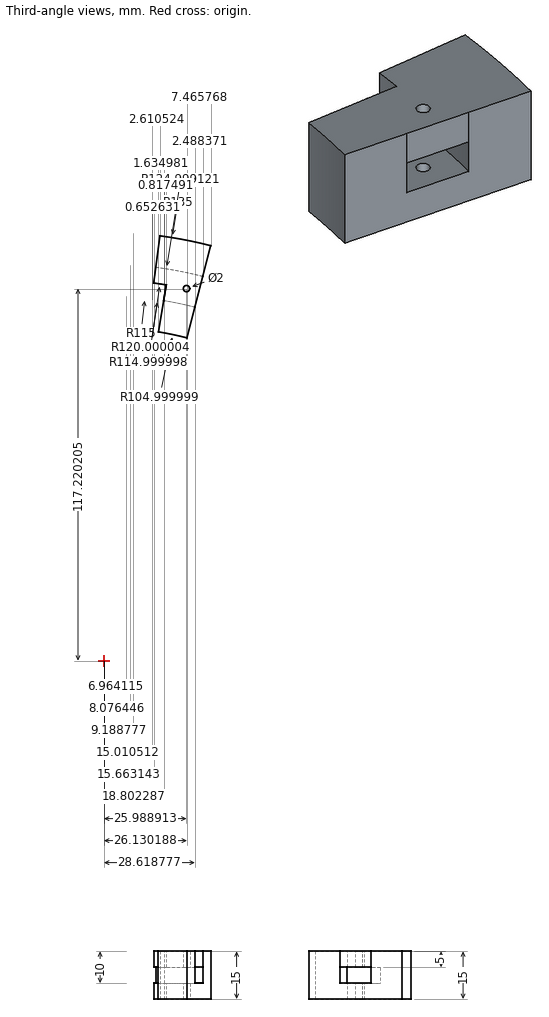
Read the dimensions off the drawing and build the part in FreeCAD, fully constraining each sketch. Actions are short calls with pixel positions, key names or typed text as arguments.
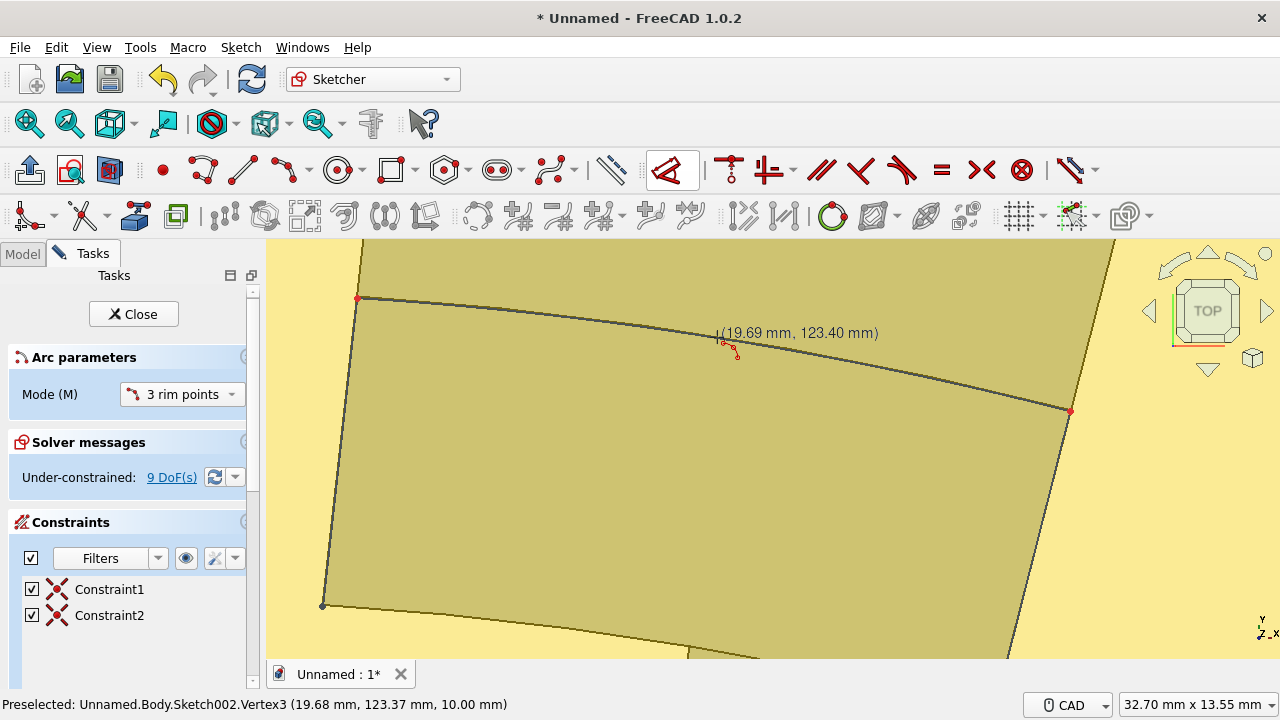
click(323, 607)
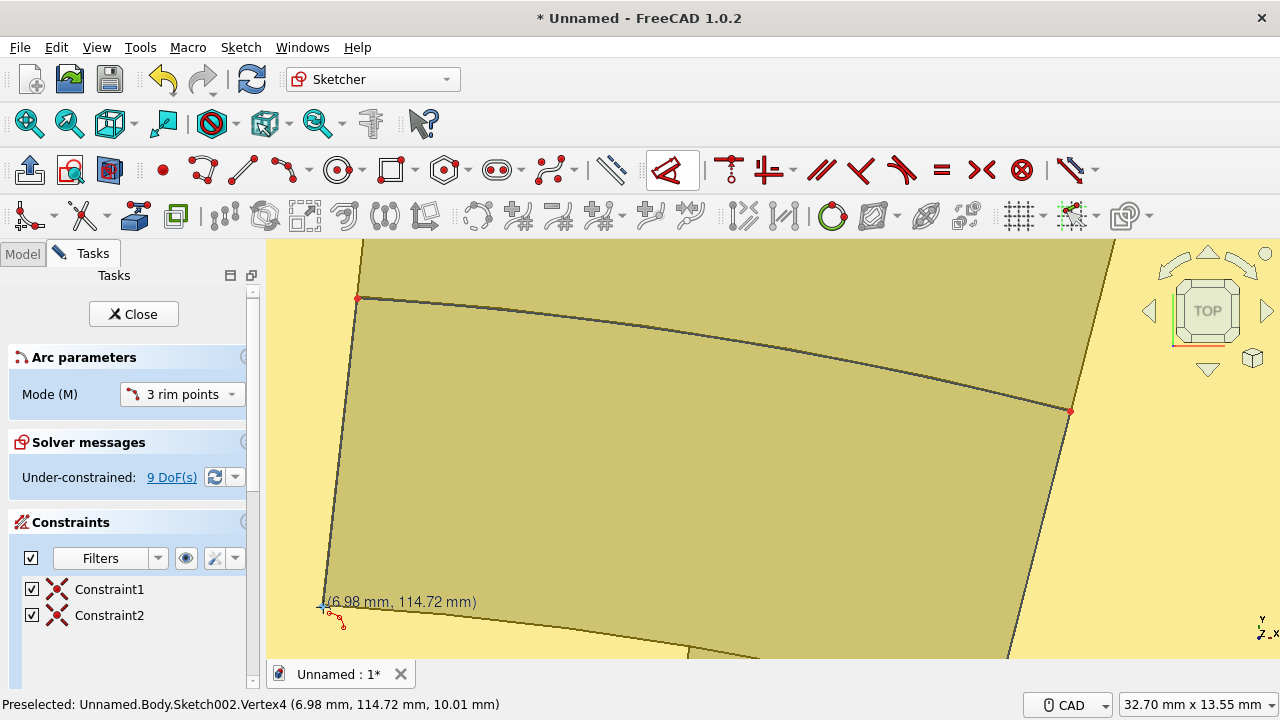
scroll(720, 338, down, 2)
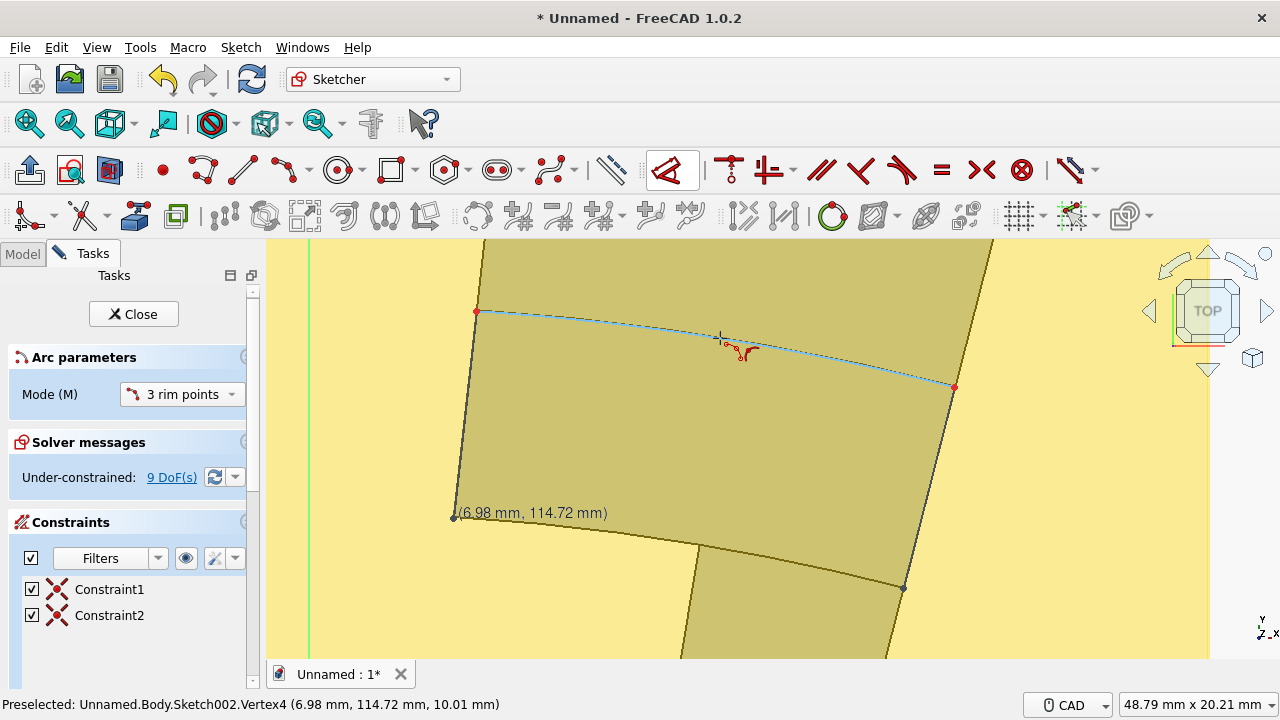
click(904, 588)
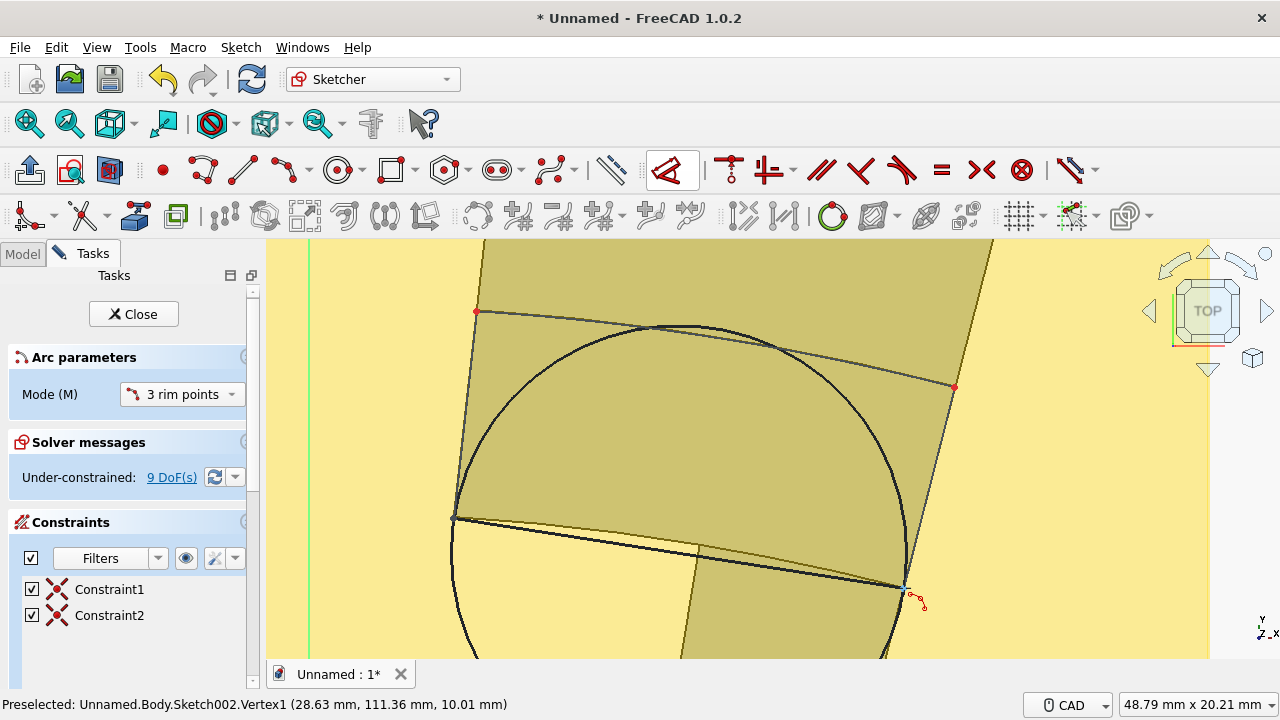
scroll(680, 542, up, 2)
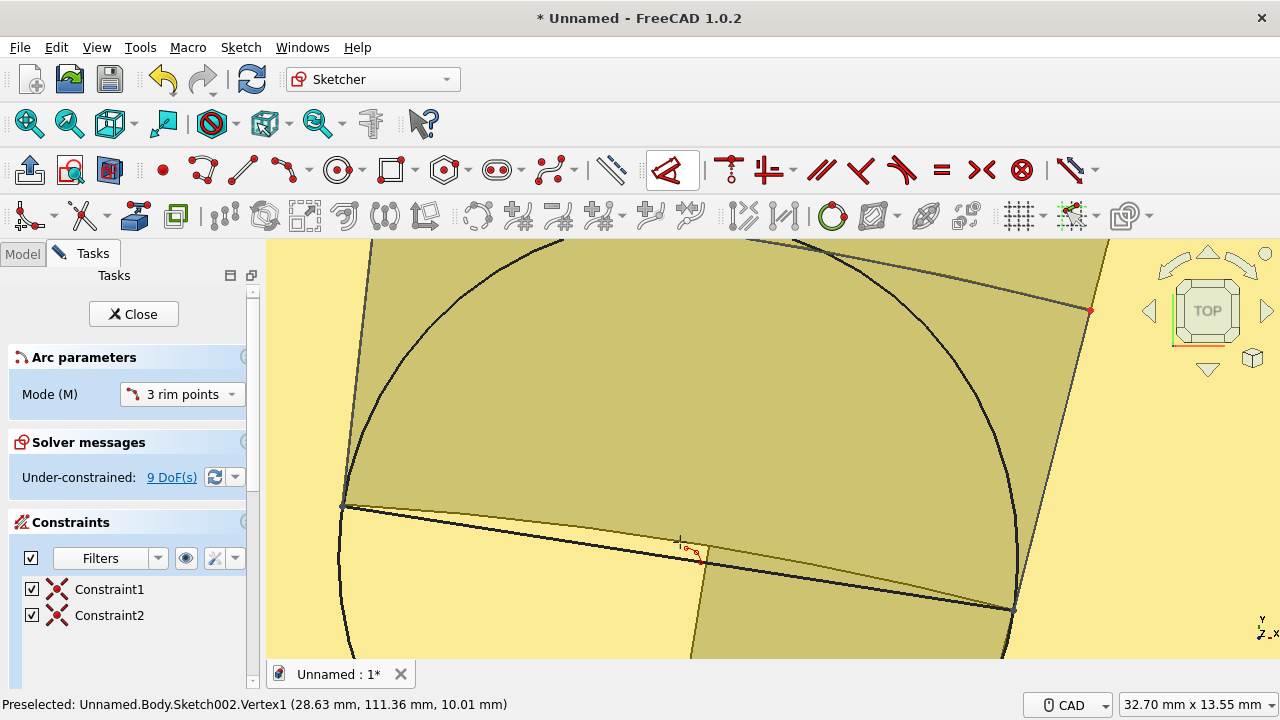
click(680, 541)
key(Escape)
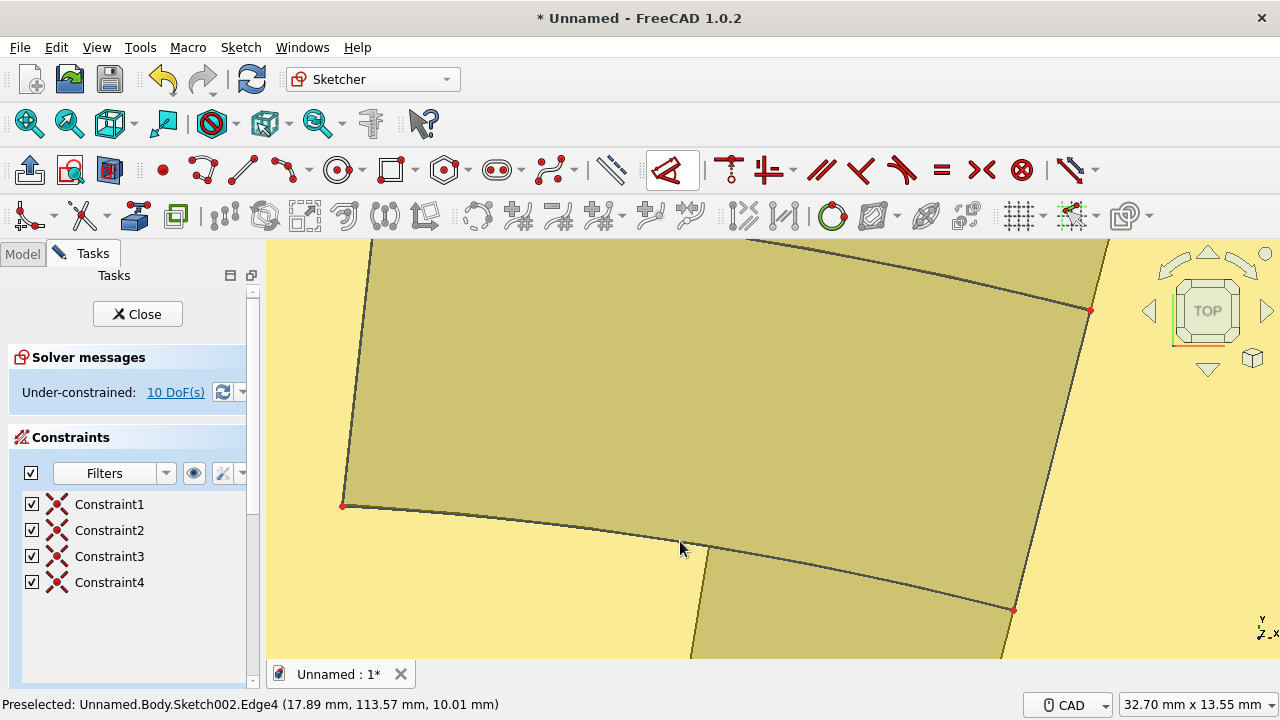
click(949, 277)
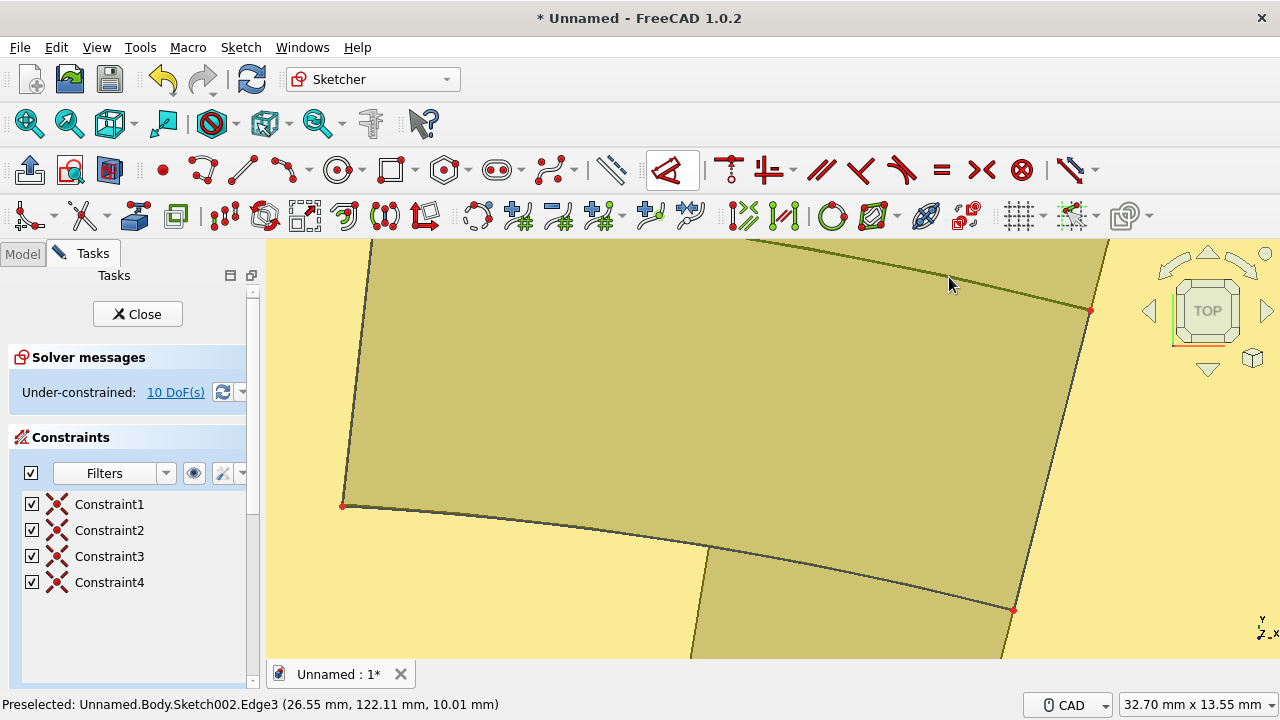
click(815, 566)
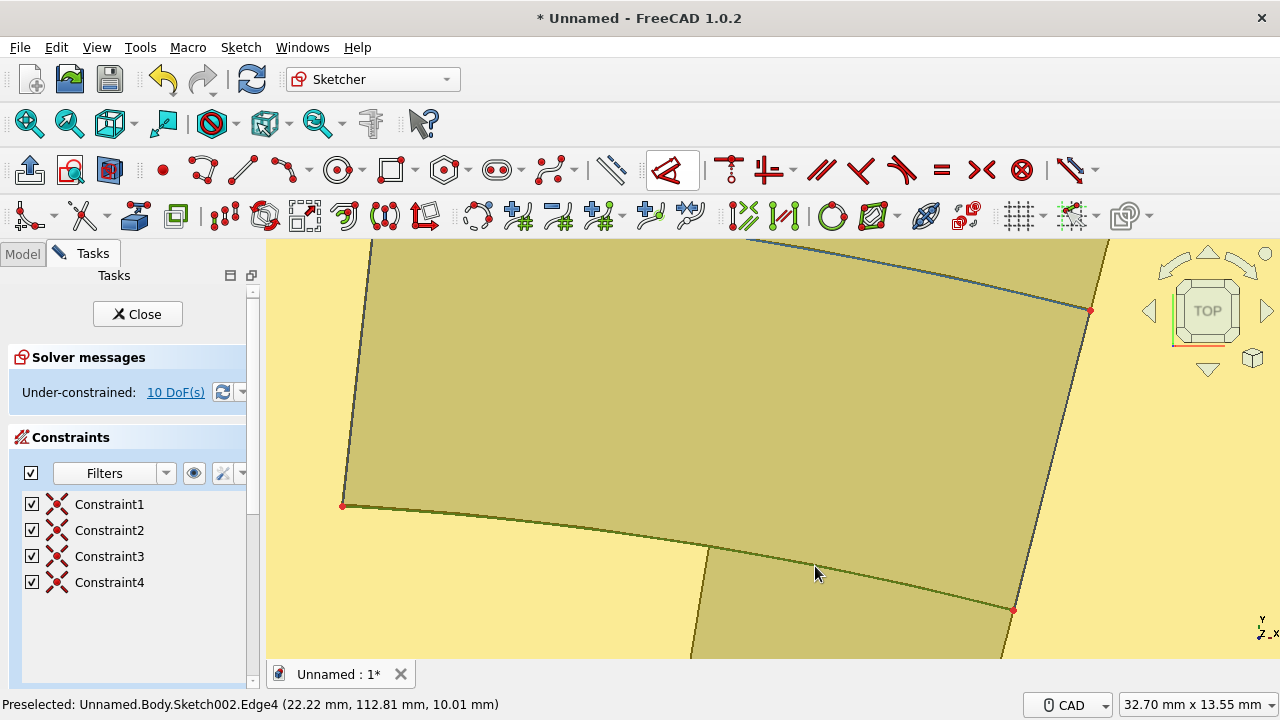
click(730, 170)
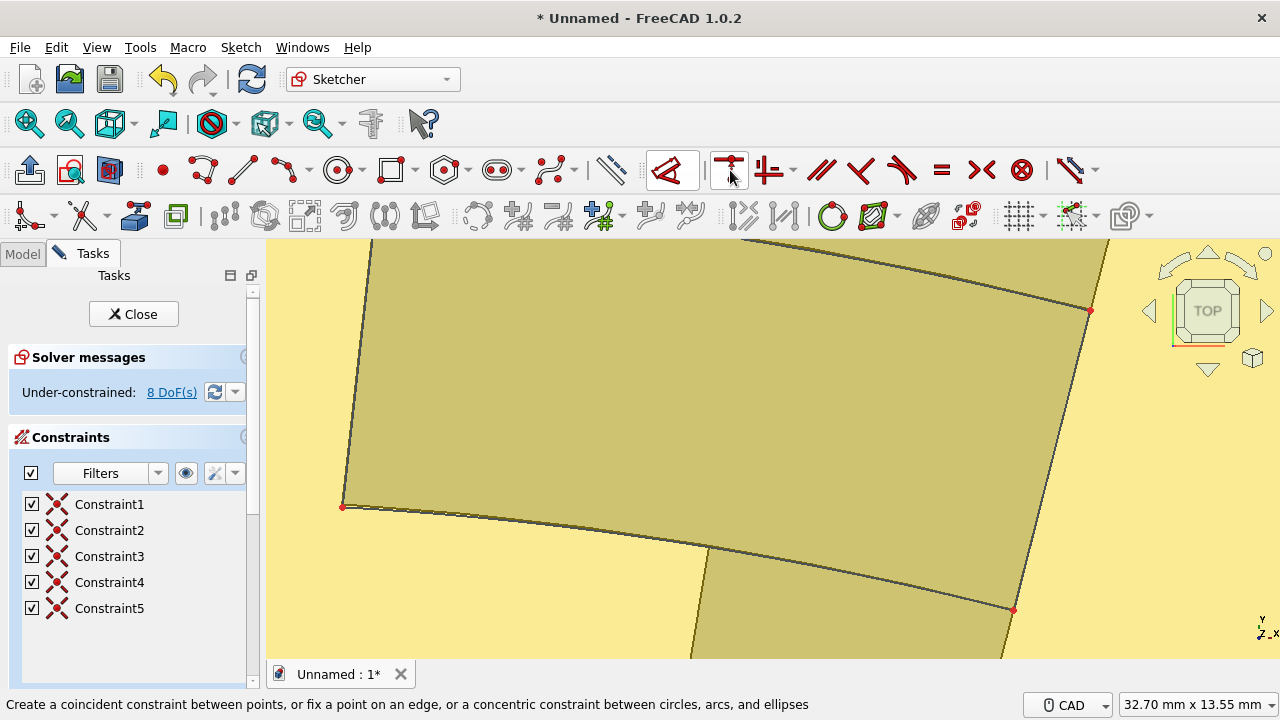
scroll(680, 543, down, 2)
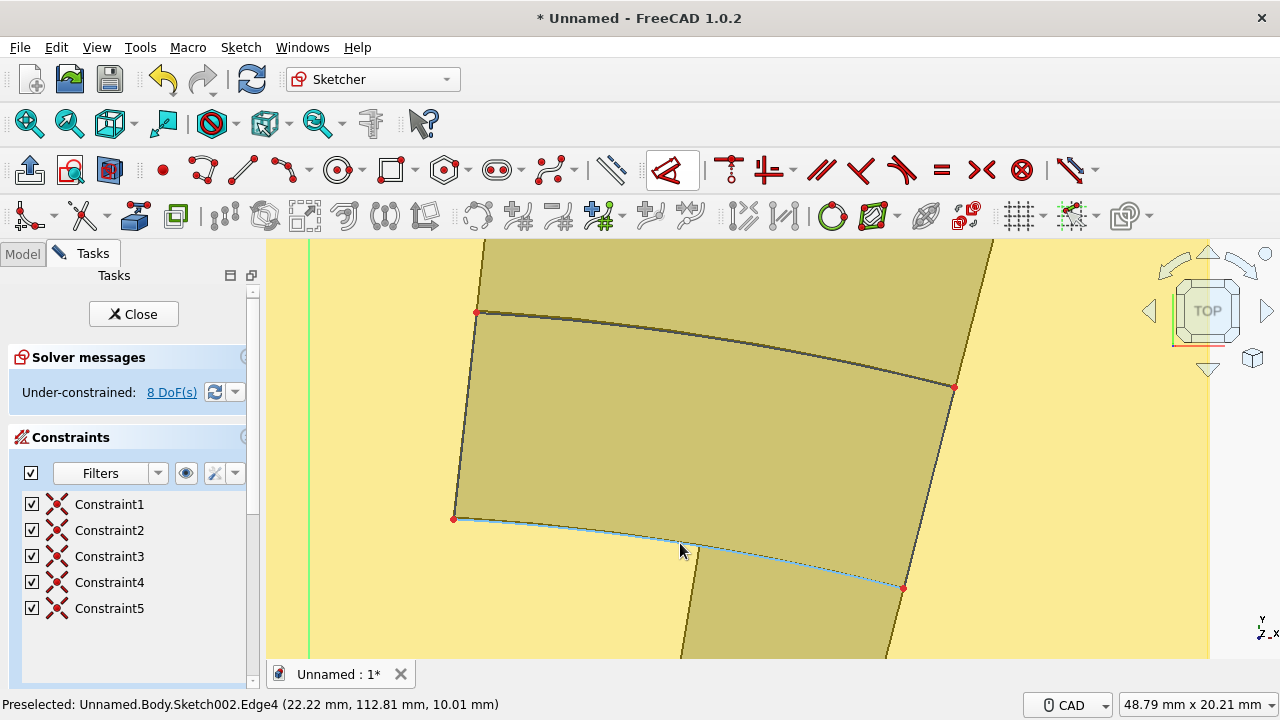
scroll(711, 334, down, 12)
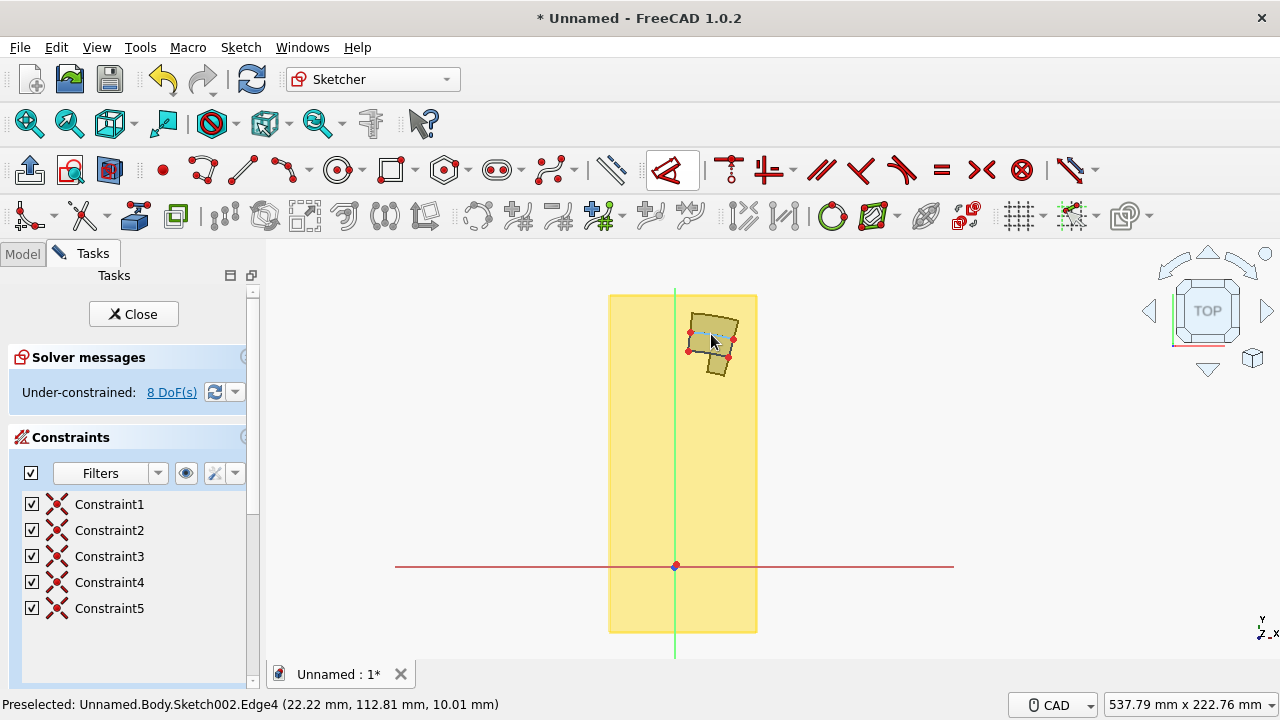
drag(665, 554, 686, 577)